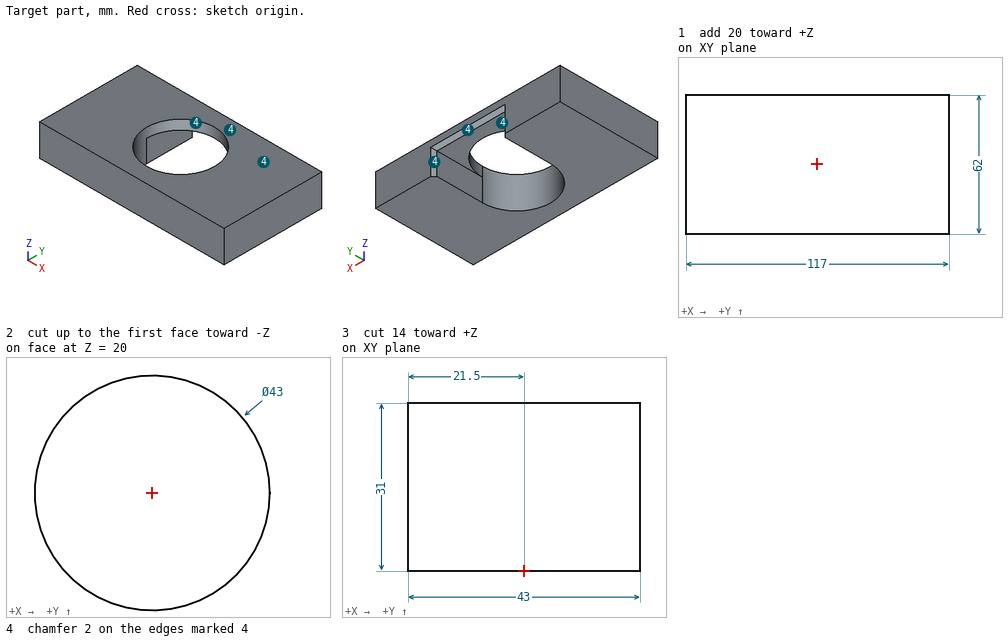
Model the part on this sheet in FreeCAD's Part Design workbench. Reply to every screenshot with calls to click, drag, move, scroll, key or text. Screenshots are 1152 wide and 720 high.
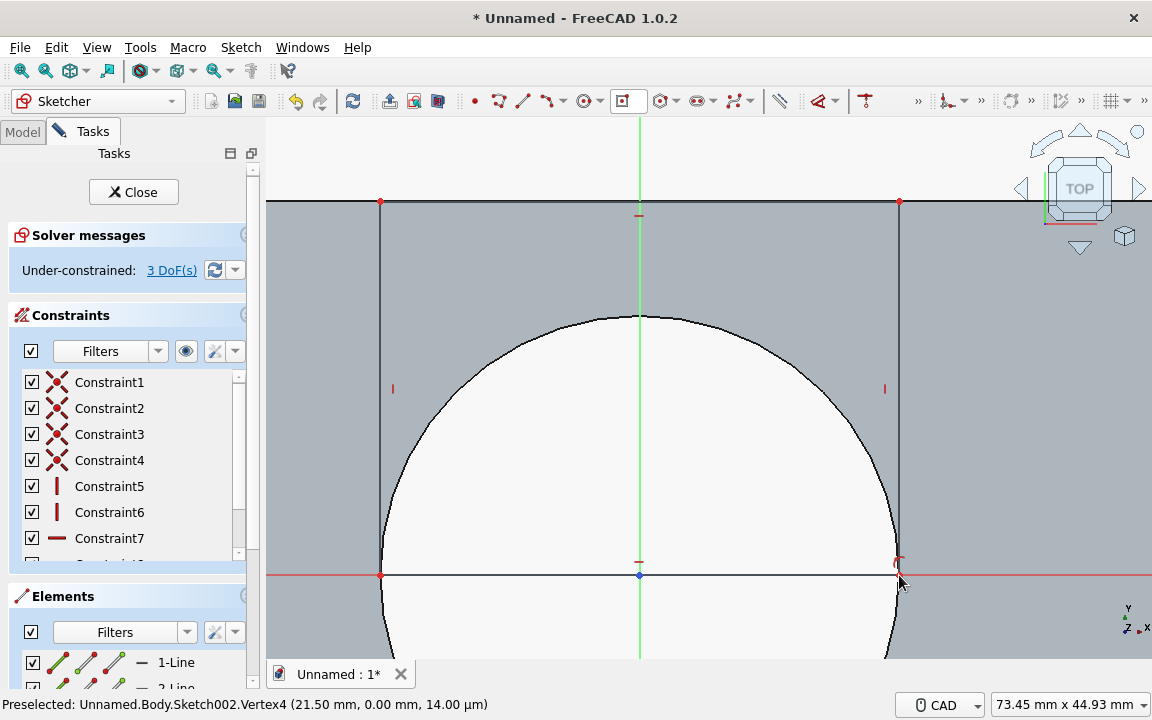
key(d)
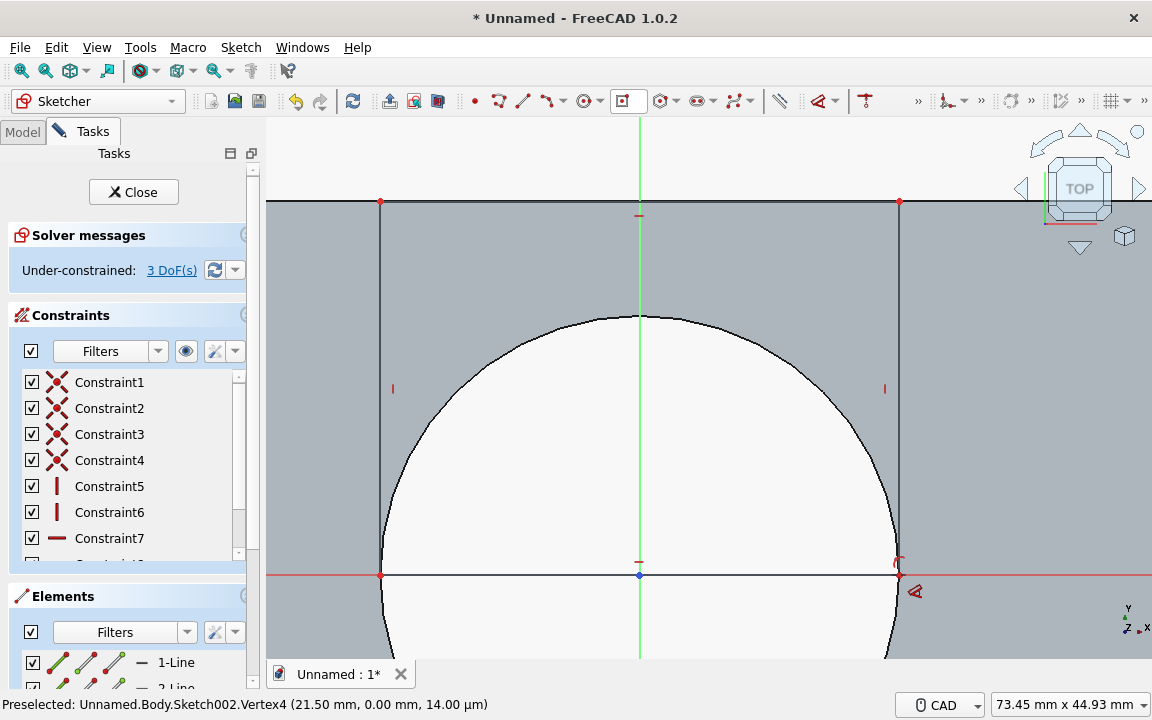
click(380, 314)
click(346, 389)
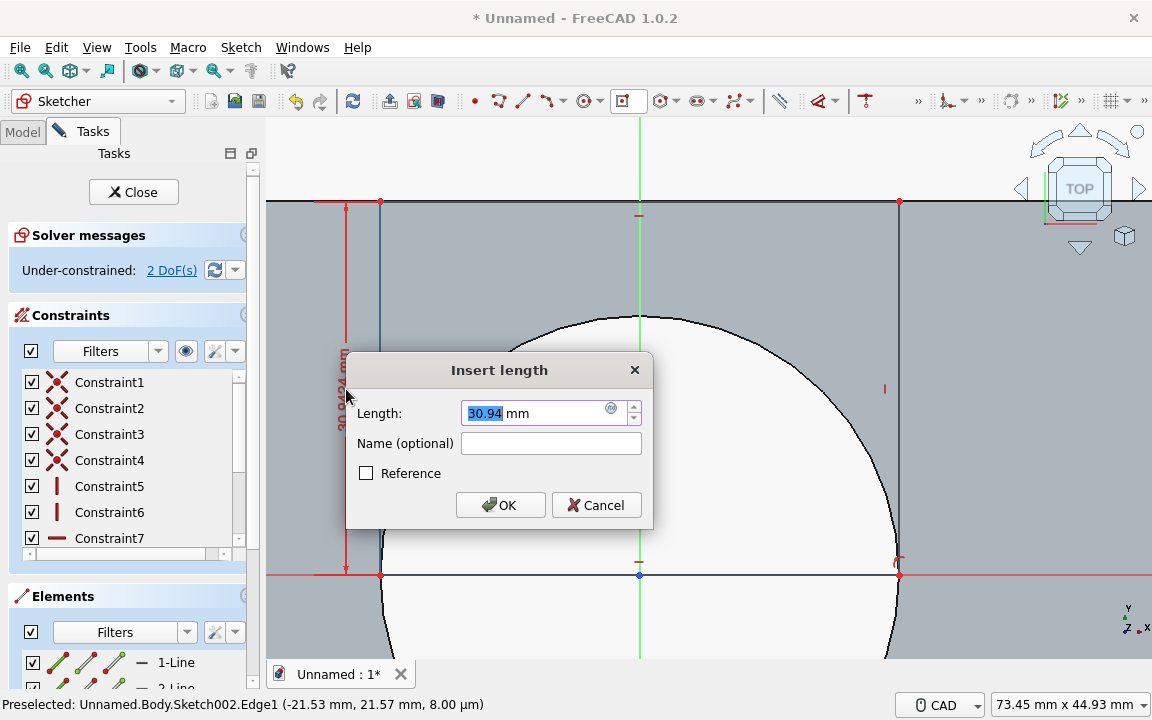
text(31)
key(Return)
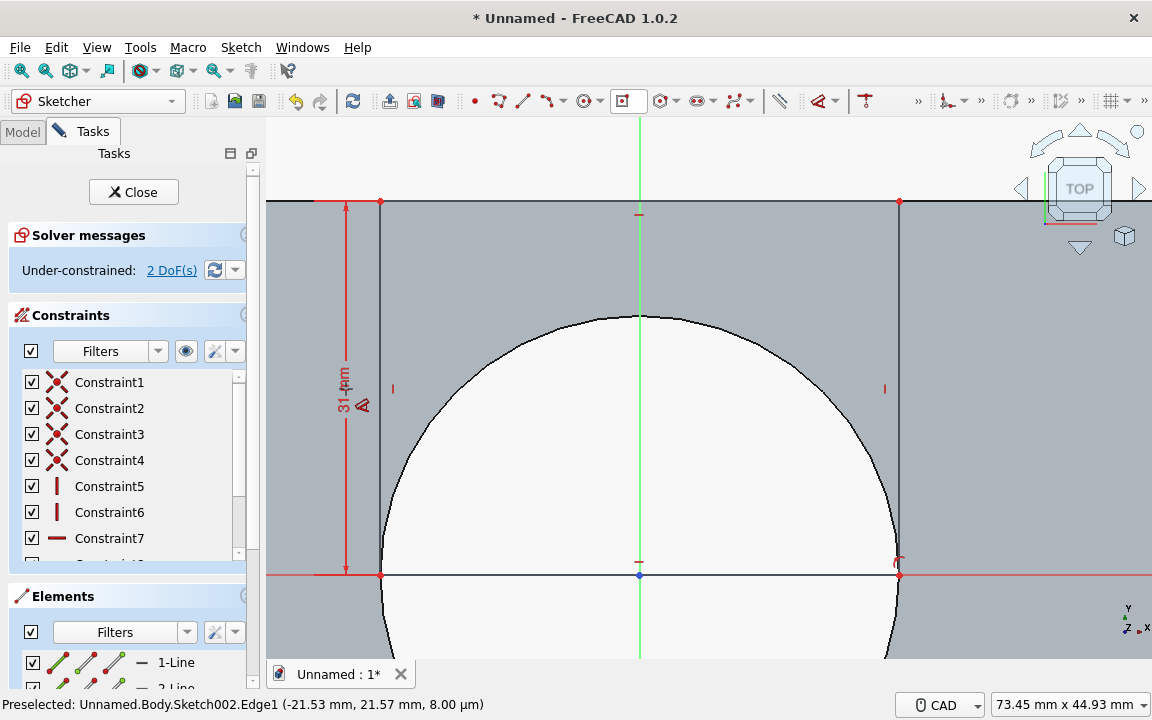
click(536, 575)
click(520, 609)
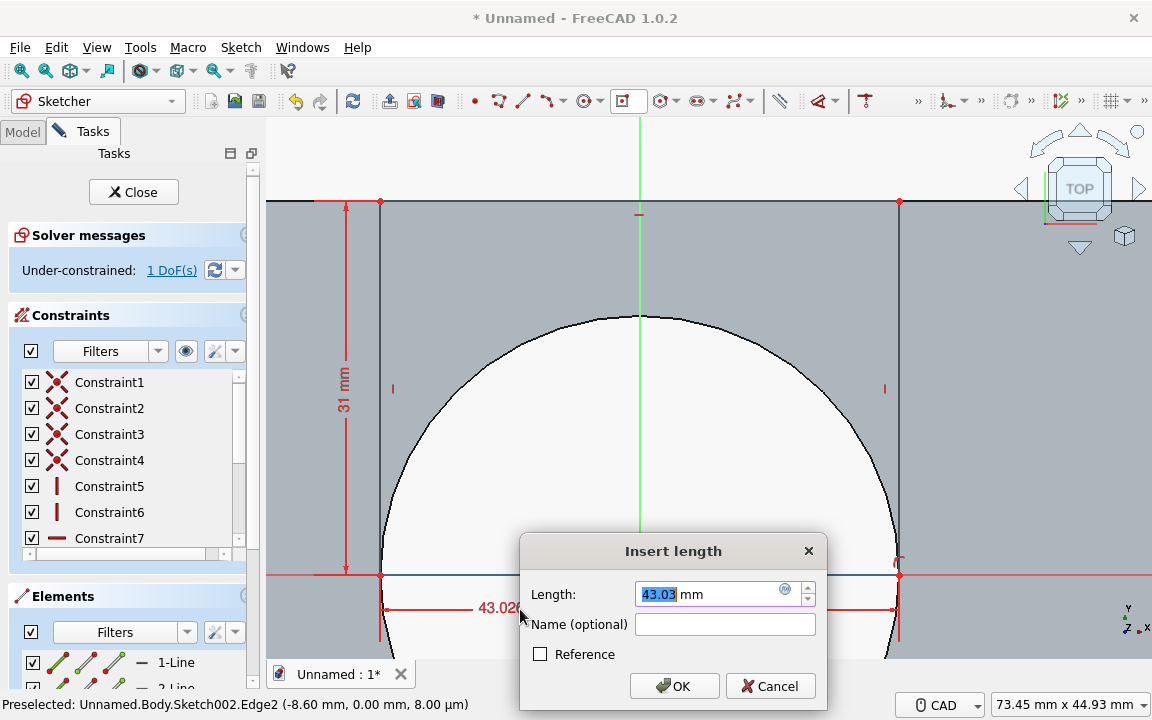
text(43)
key(Return)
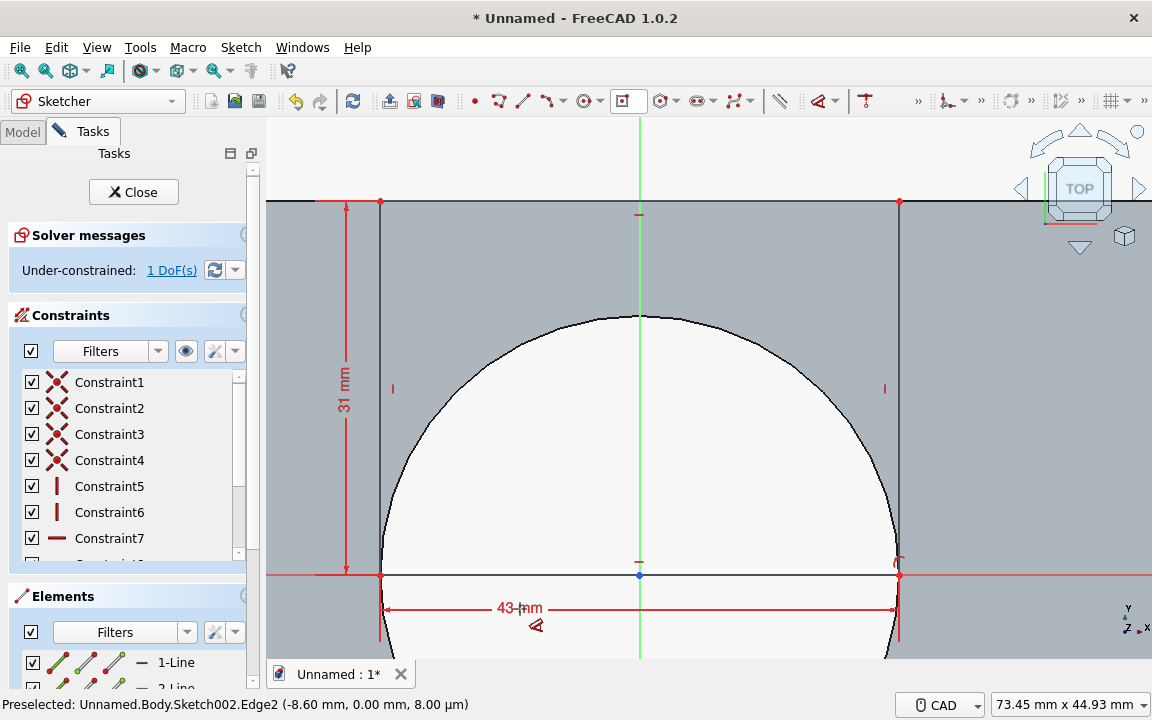
click(380, 201)
click(419, 609)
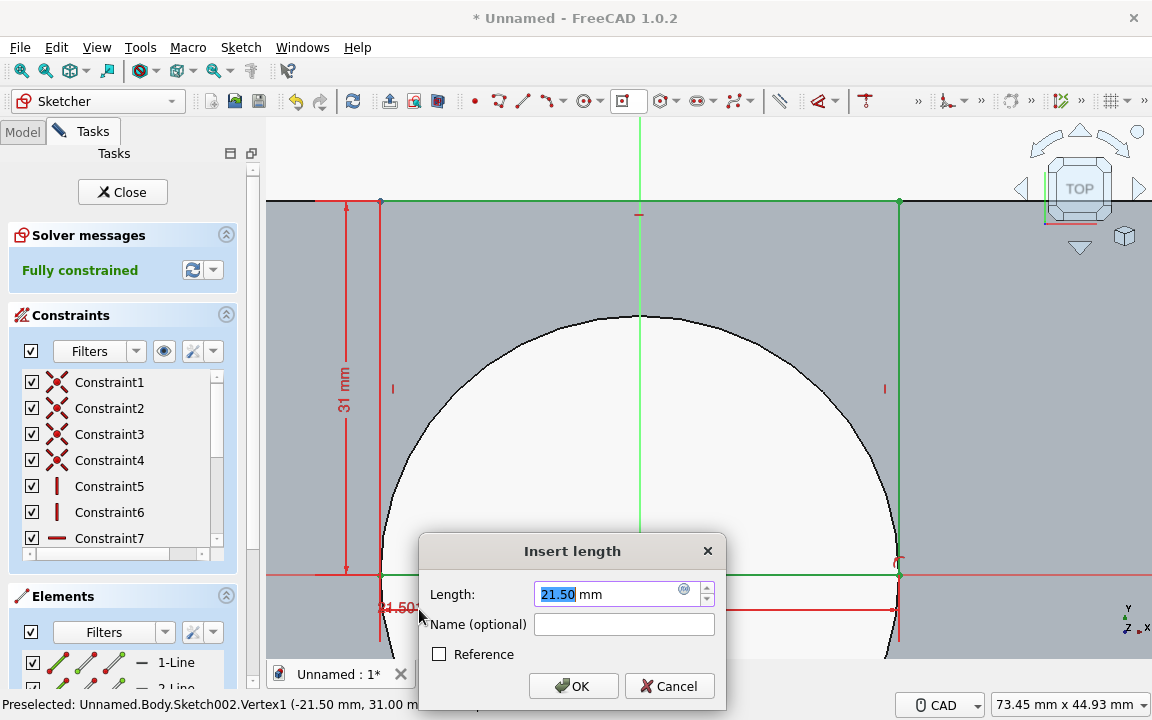
text(21.5)
key(Return)
key(Escape)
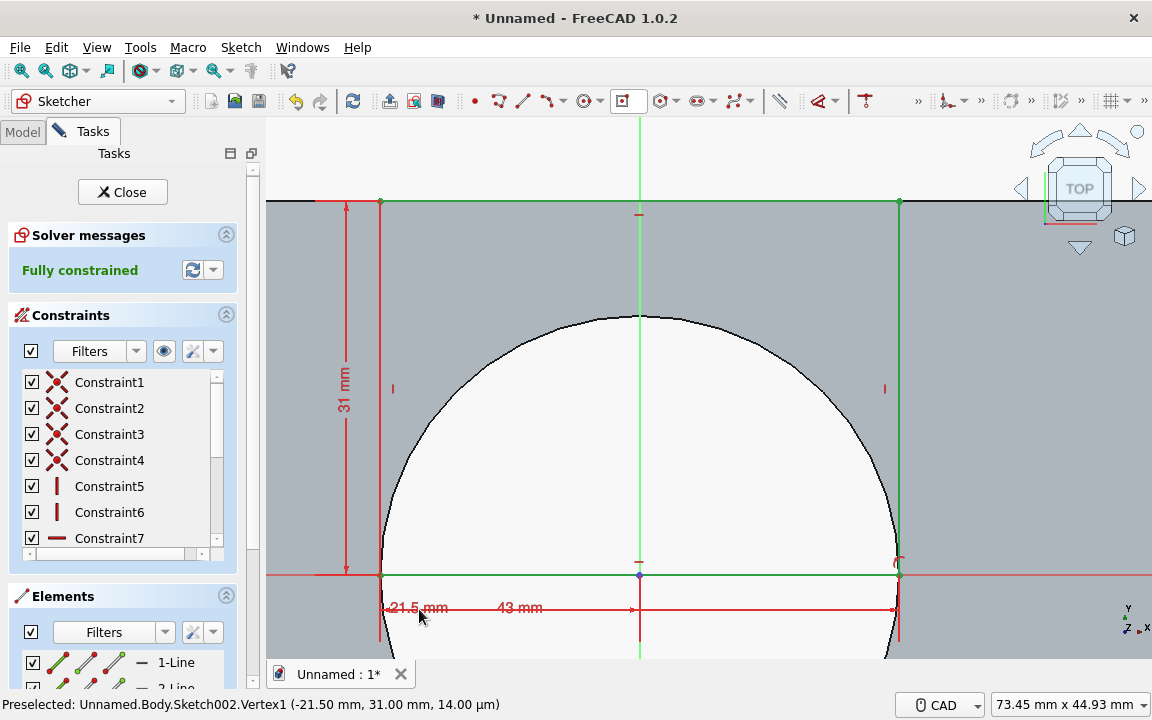
click(123, 192)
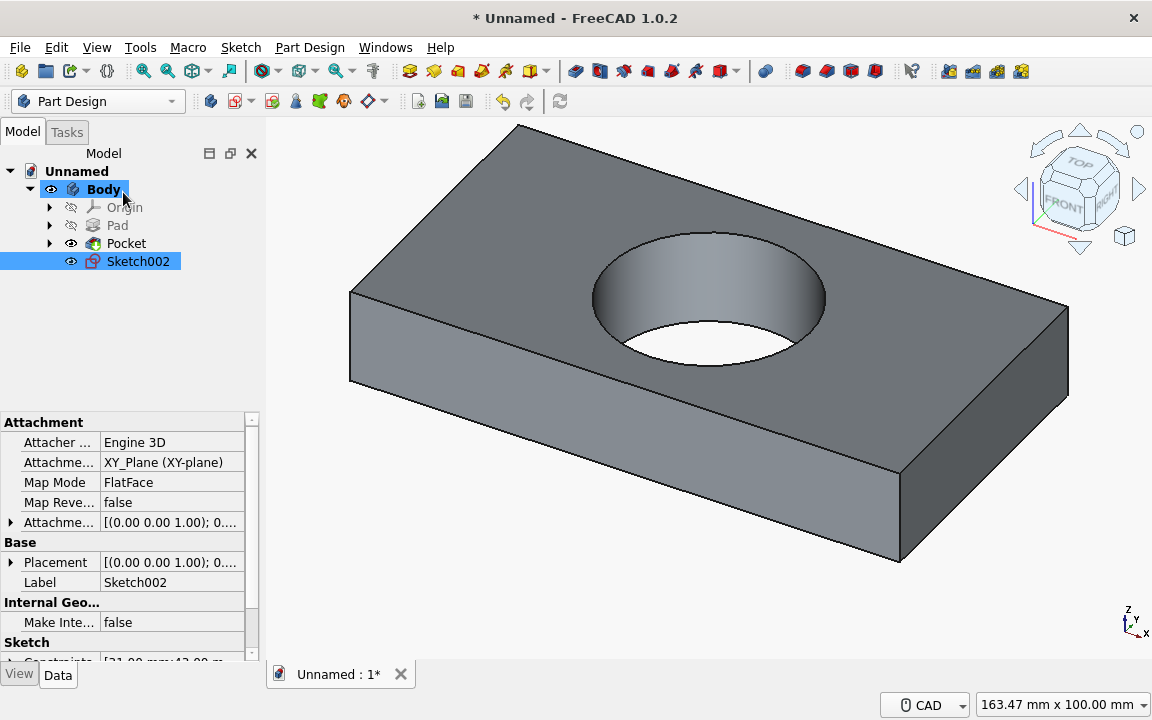
click(576, 72)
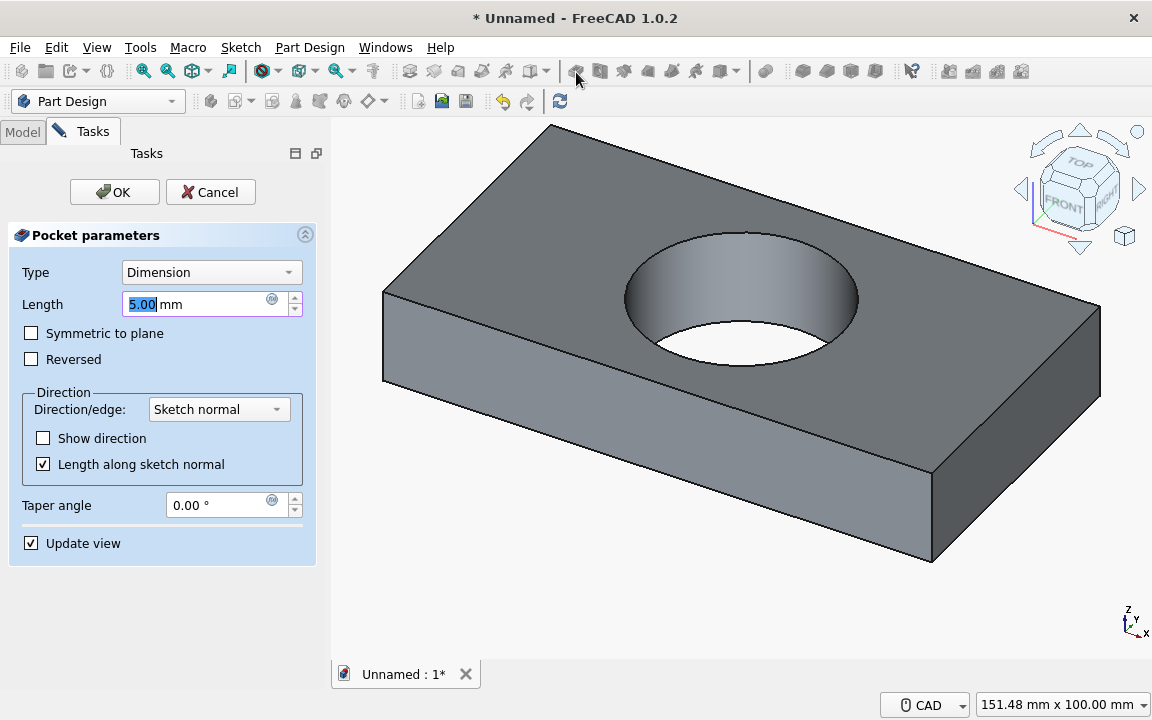
text(14)
key(Tab)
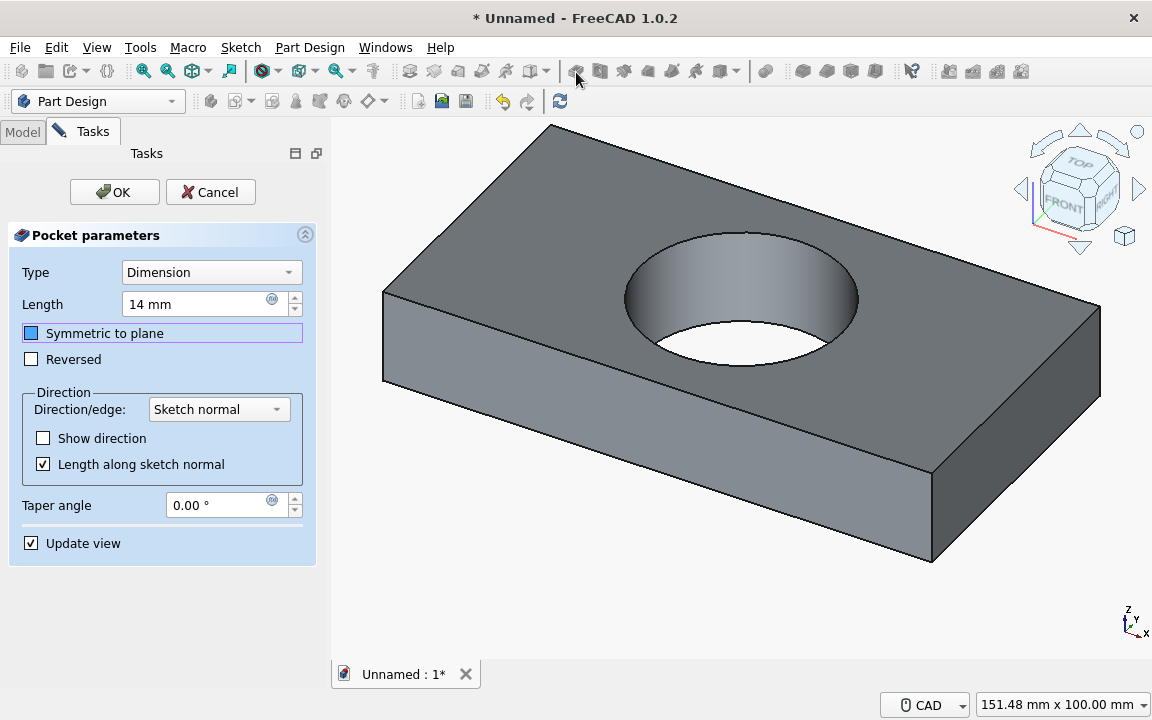
click(30, 359)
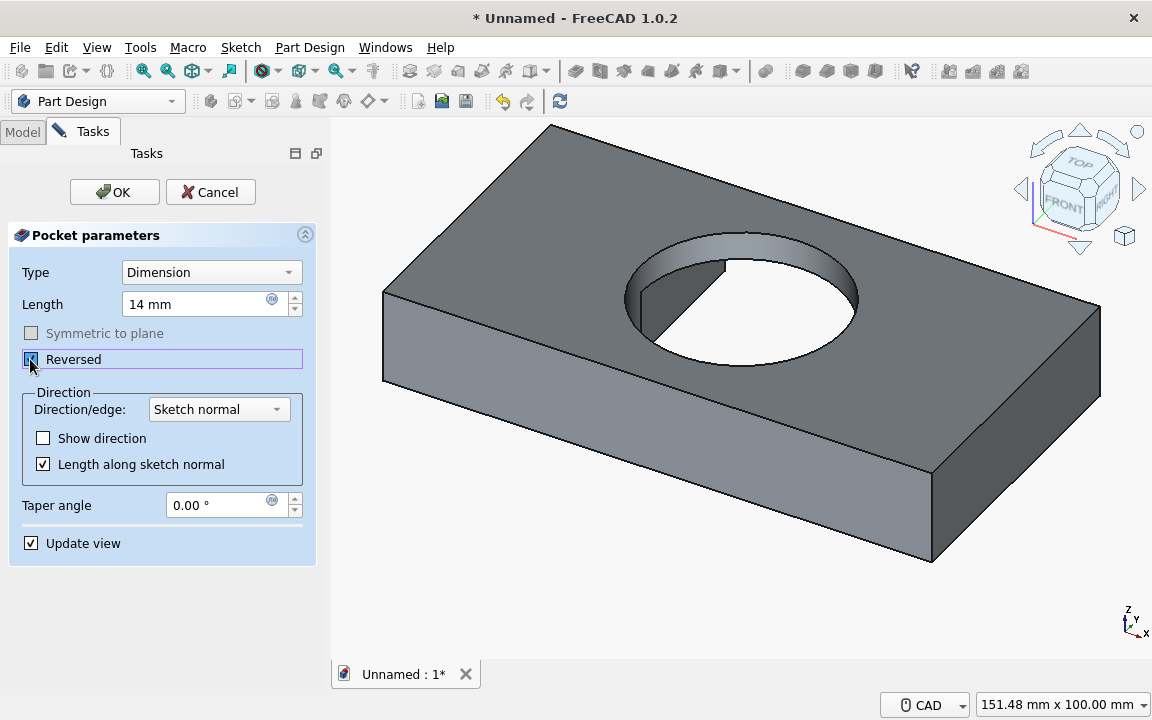
click(115, 192)